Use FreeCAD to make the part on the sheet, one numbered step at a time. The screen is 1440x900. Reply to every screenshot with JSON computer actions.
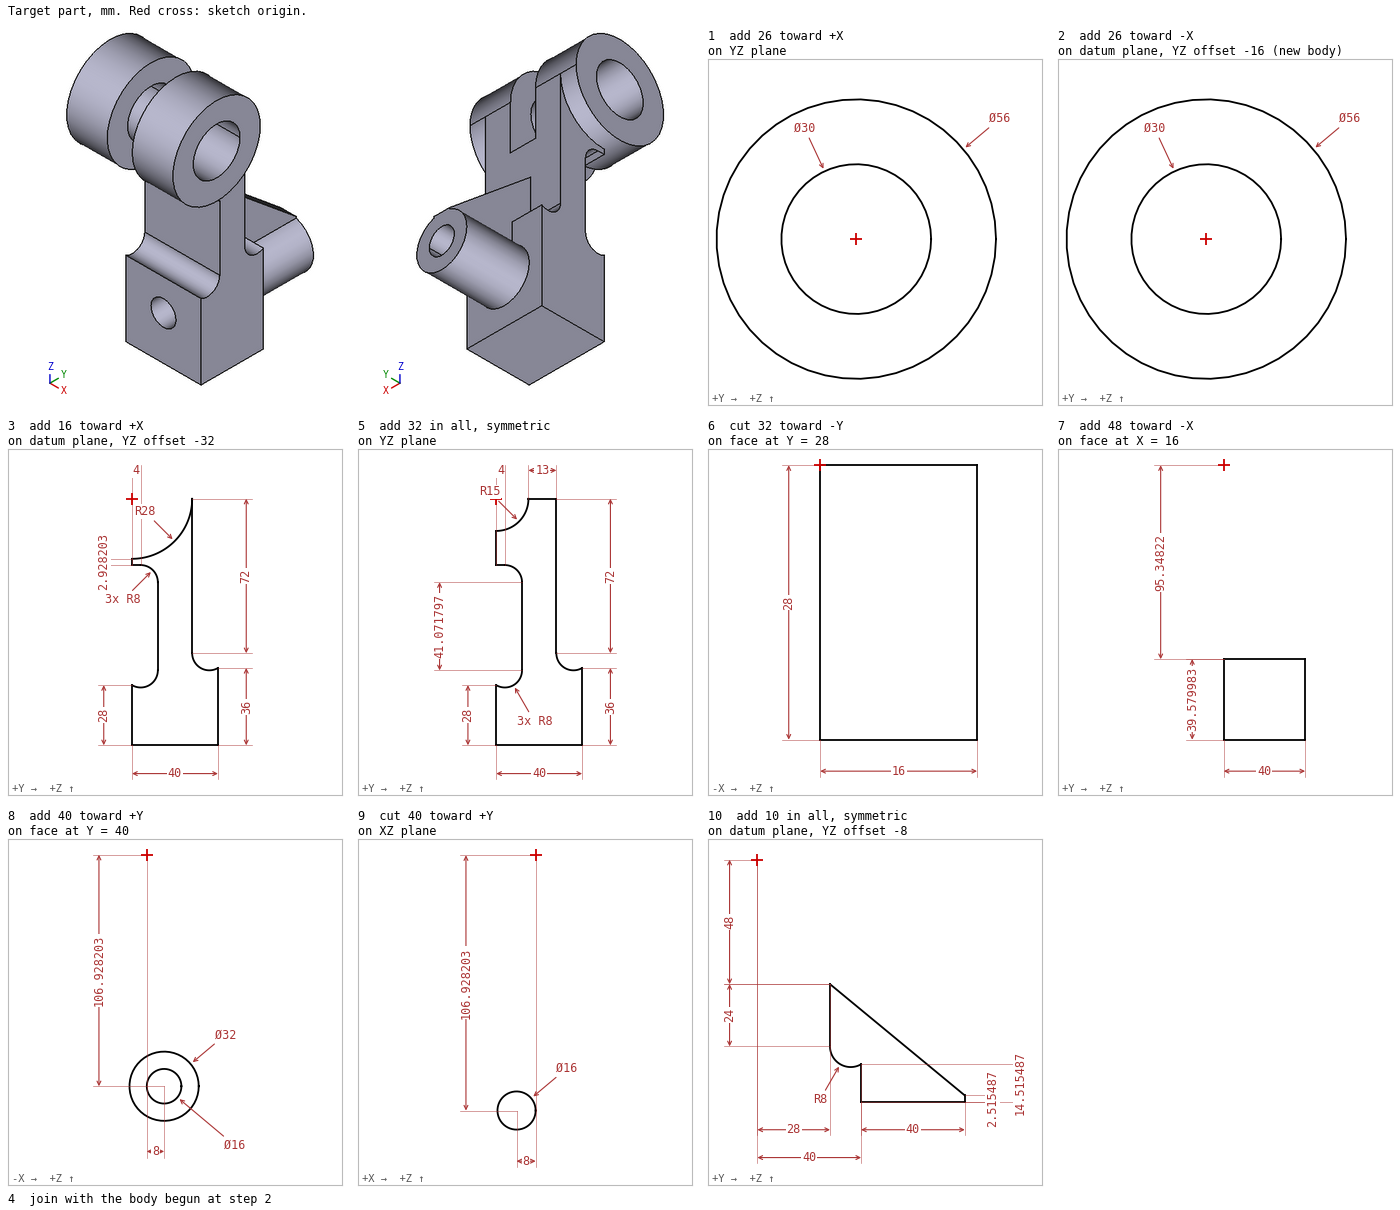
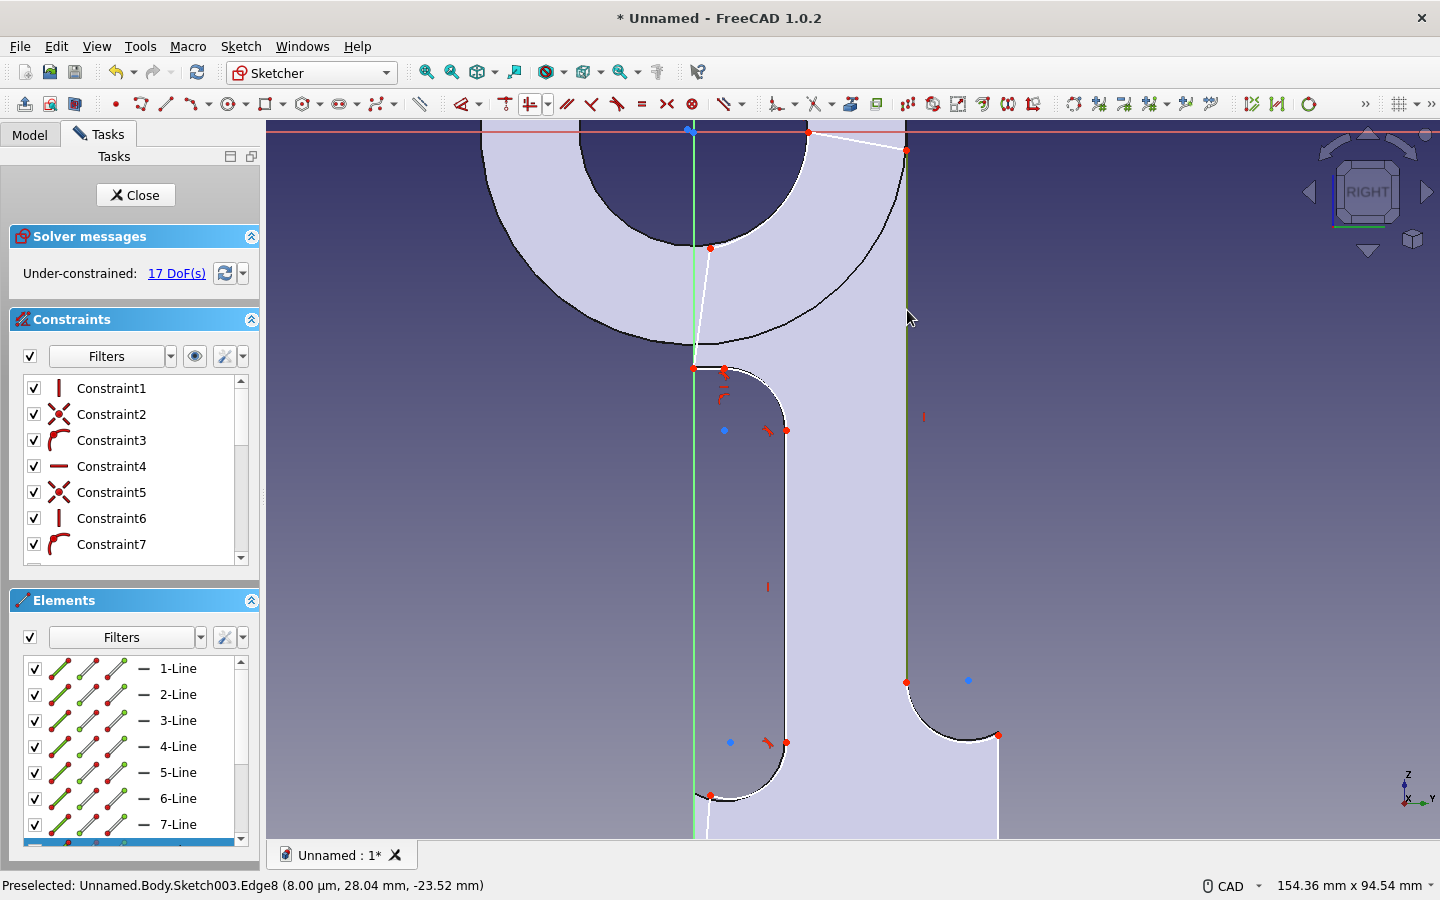
{"action": "left_click", "coordinate": [919, 718]}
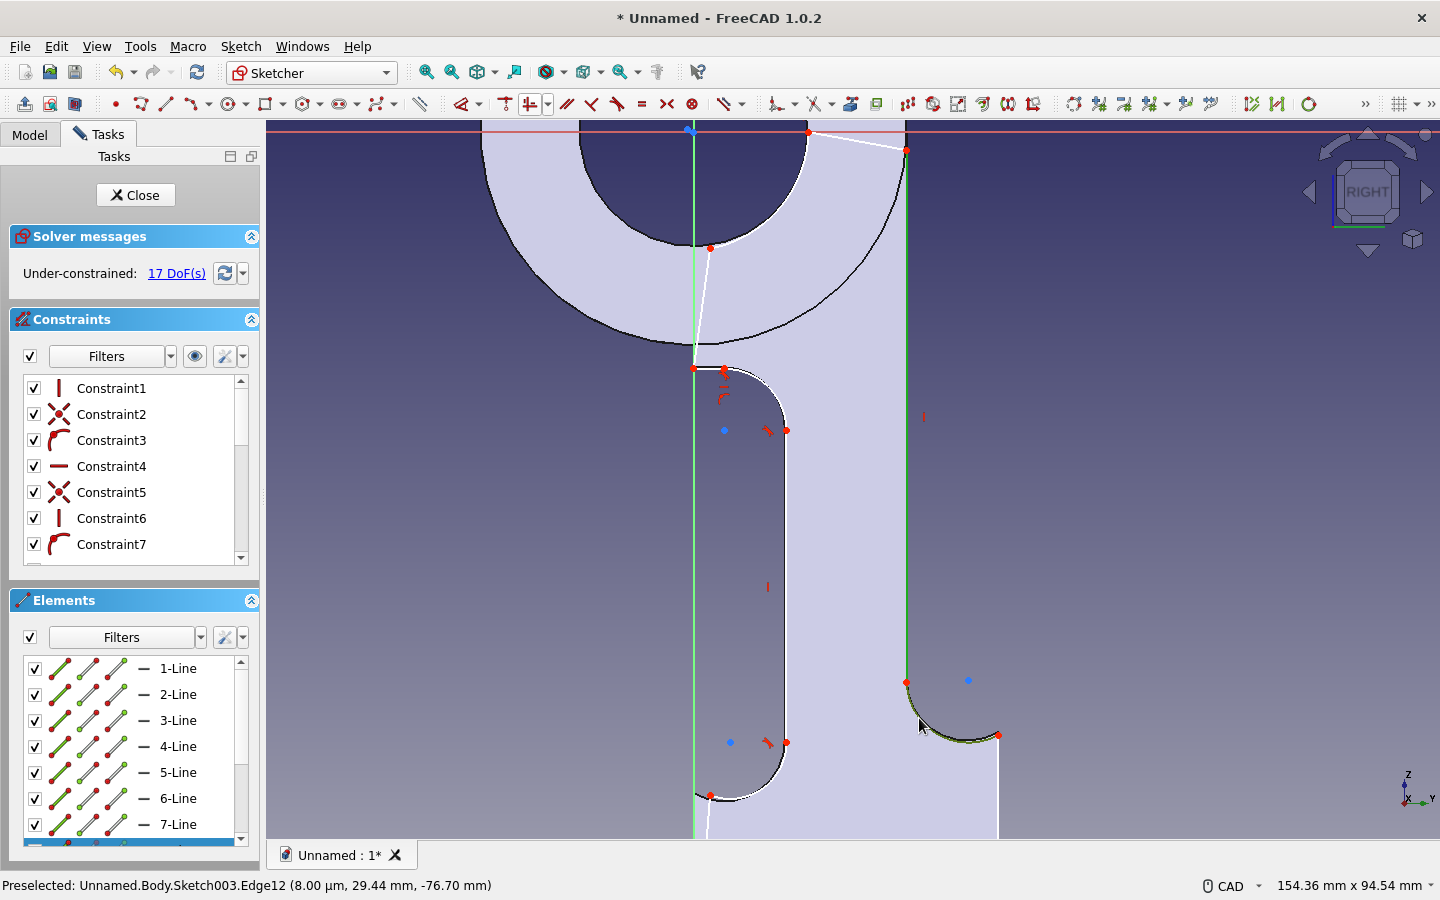
{"action": "left_click", "coordinate": [617, 104]}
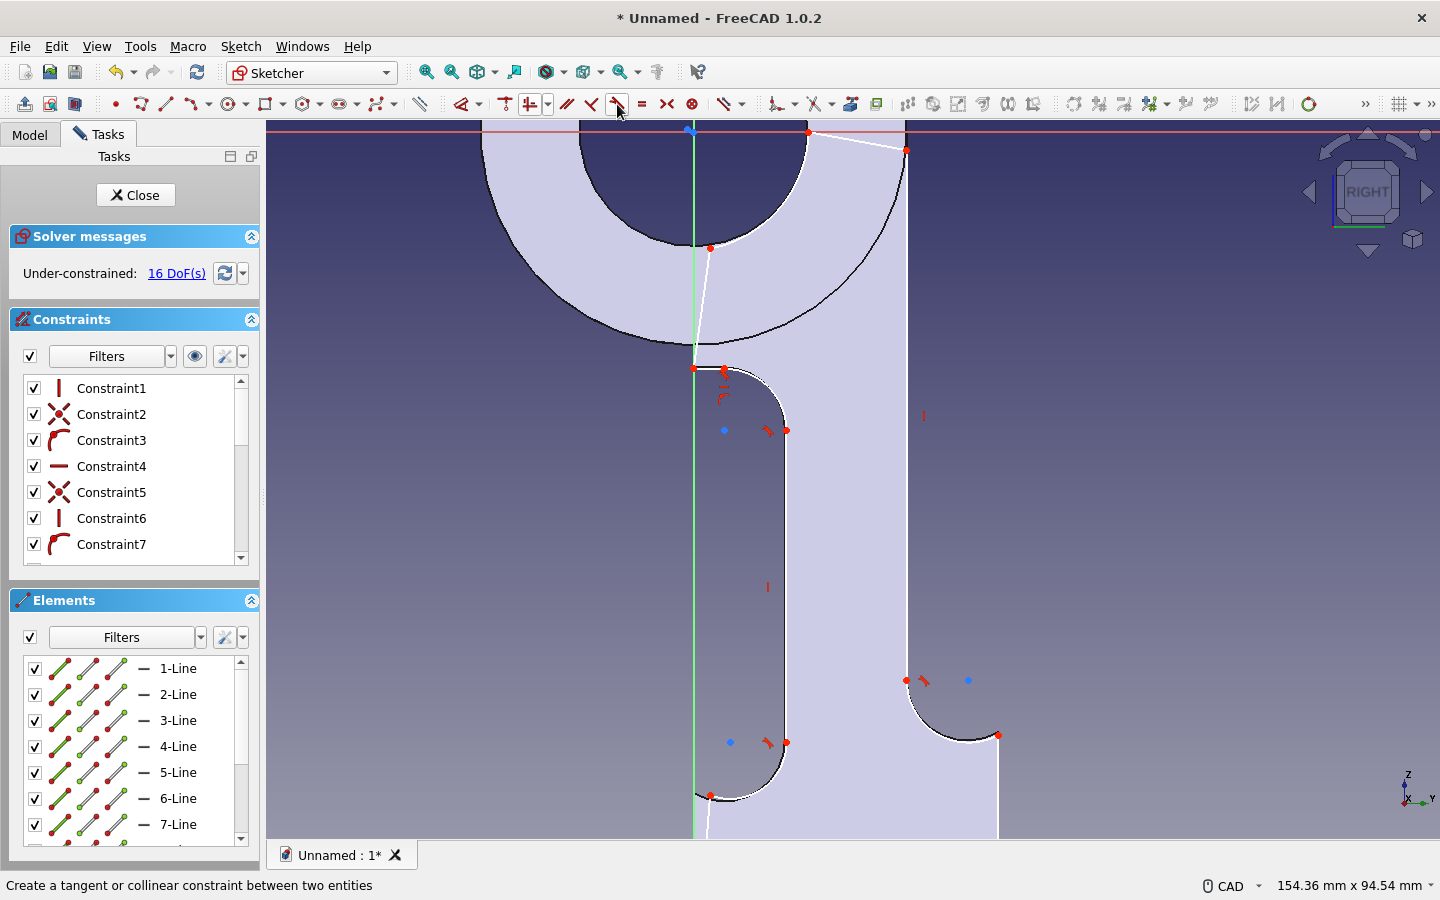
{"action": "scroll", "coordinate": [710, 370], "scroll_direction": "down", "scroll_amount": 3}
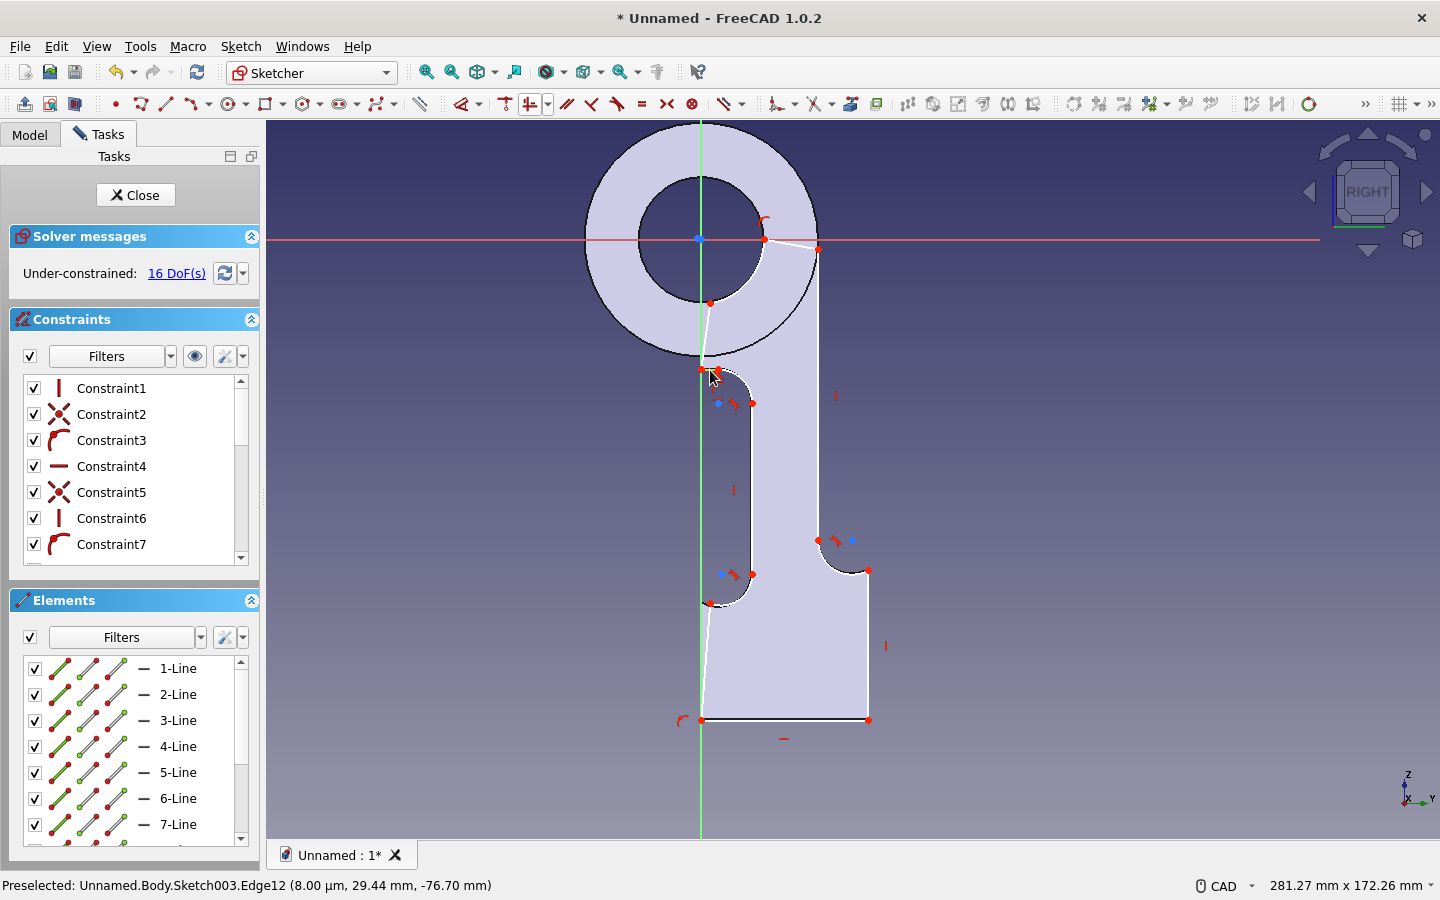
{"action": "scroll", "coordinate": [708, 639], "scroll_direction": "up", "scroll_amount": 4}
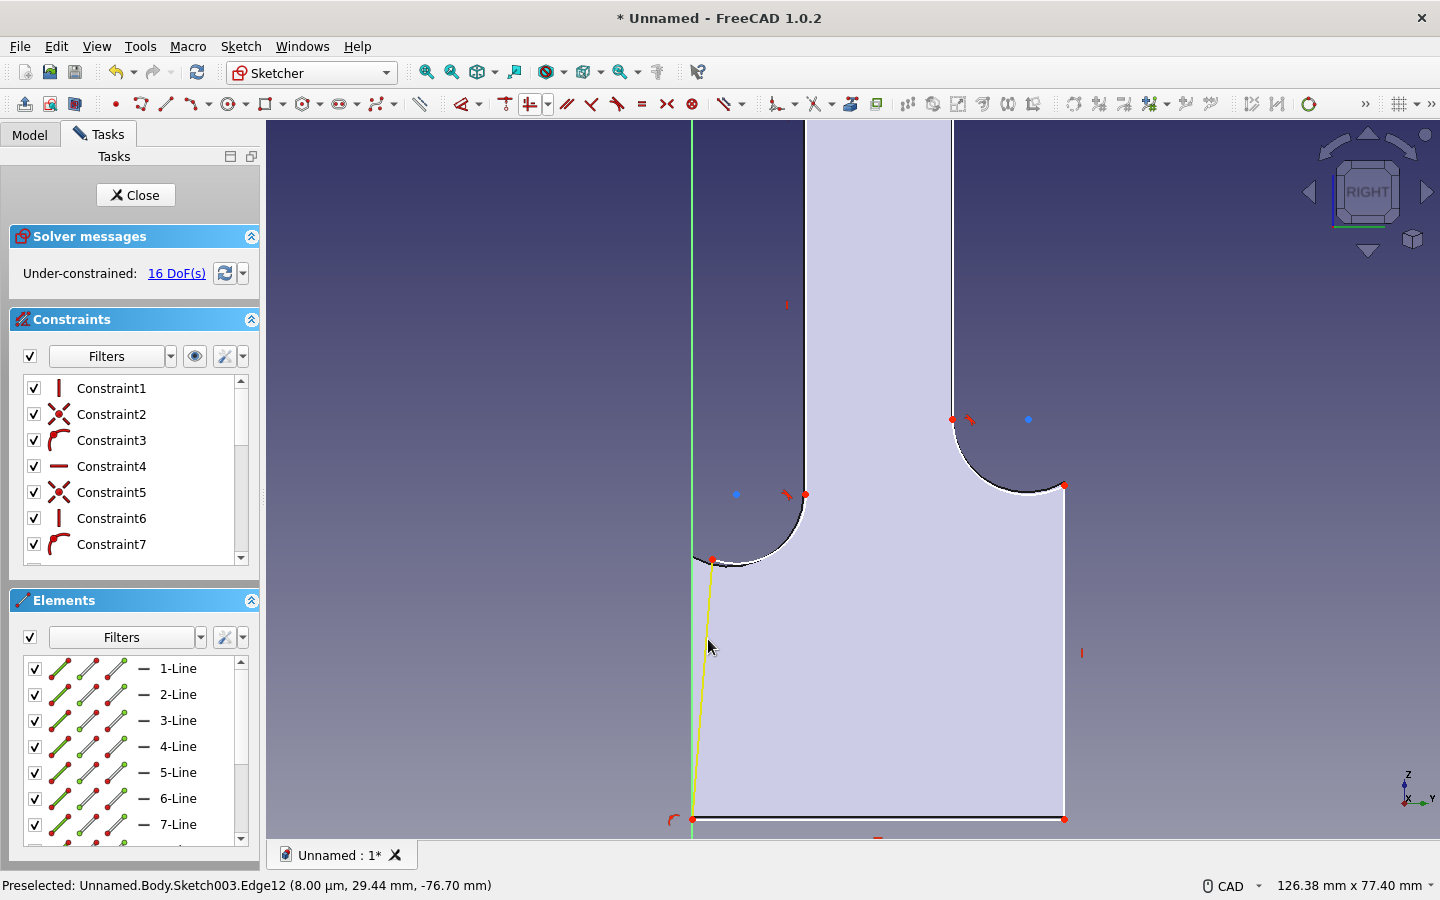
{"action": "left_click", "coordinate": [706, 637]}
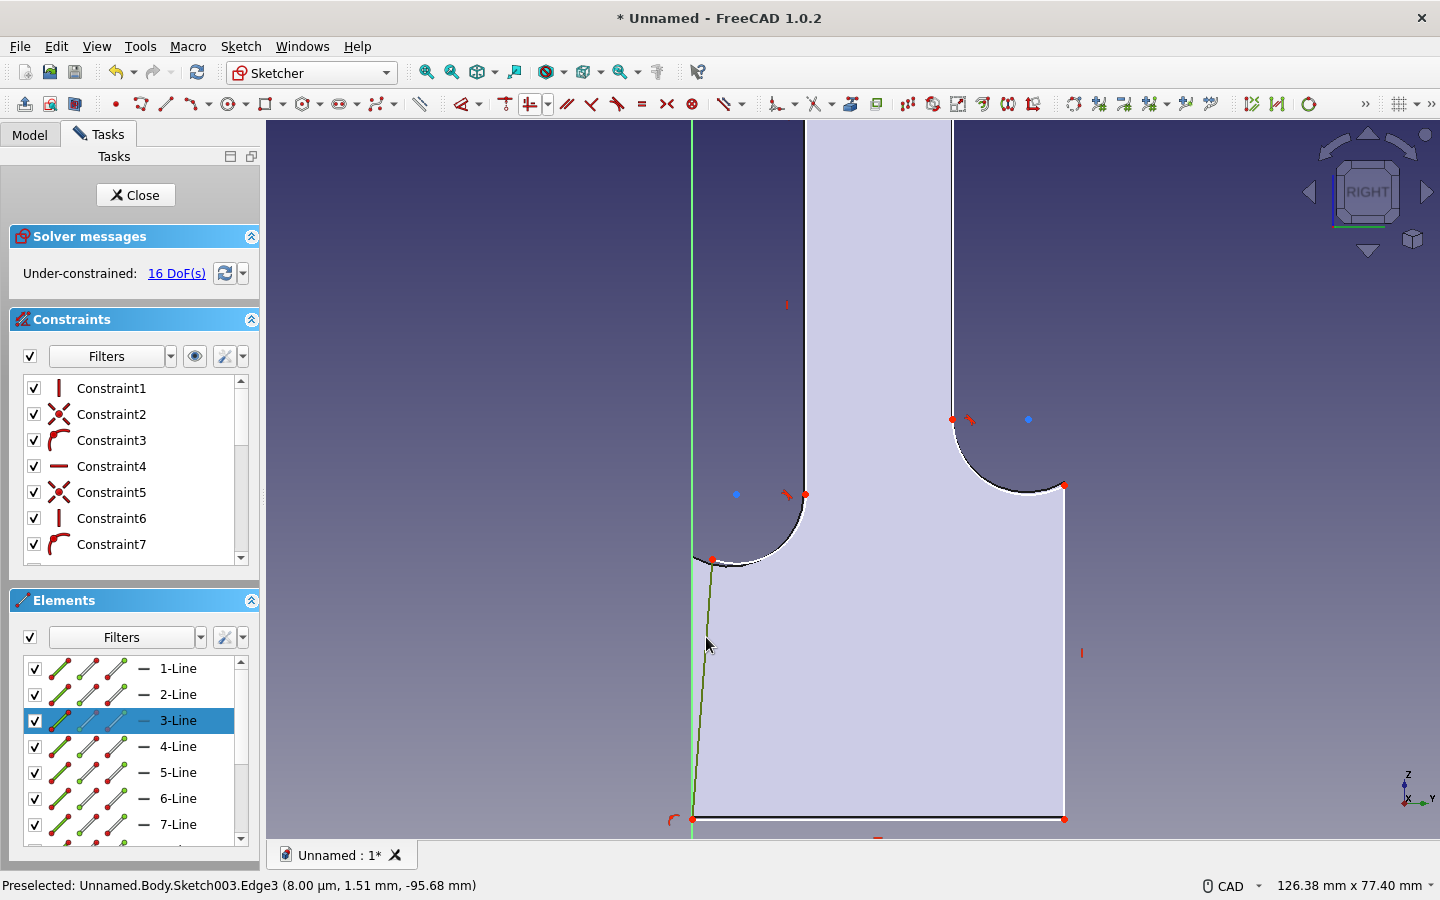
{"action": "key", "text": "v"}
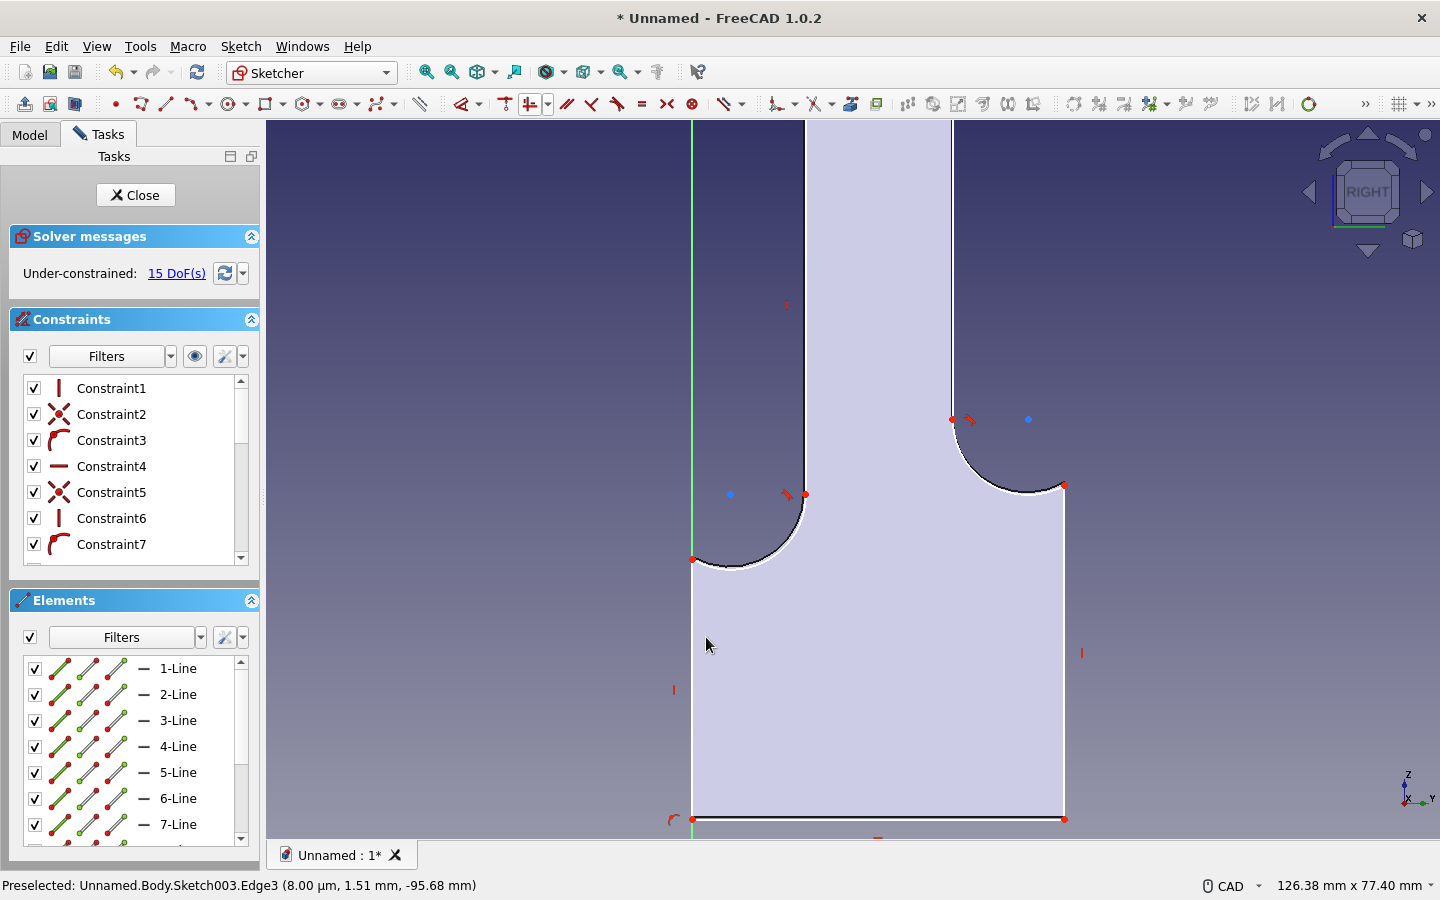
{"action": "scroll", "coordinate": [708, 640], "scroll_direction": "down", "scroll_amount": 4}